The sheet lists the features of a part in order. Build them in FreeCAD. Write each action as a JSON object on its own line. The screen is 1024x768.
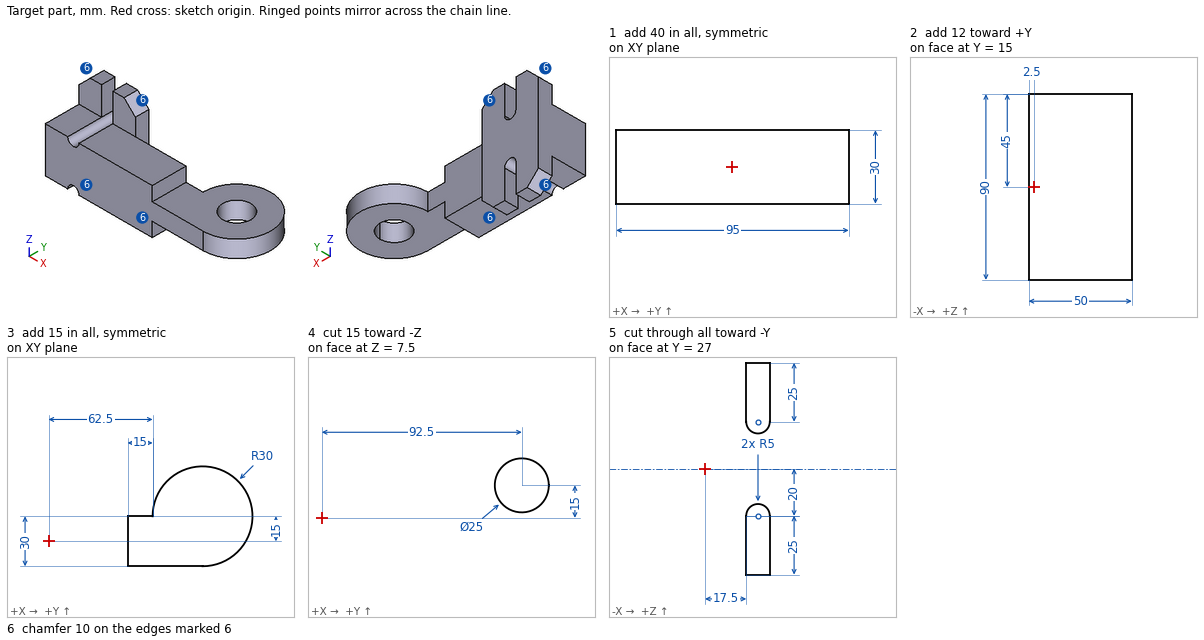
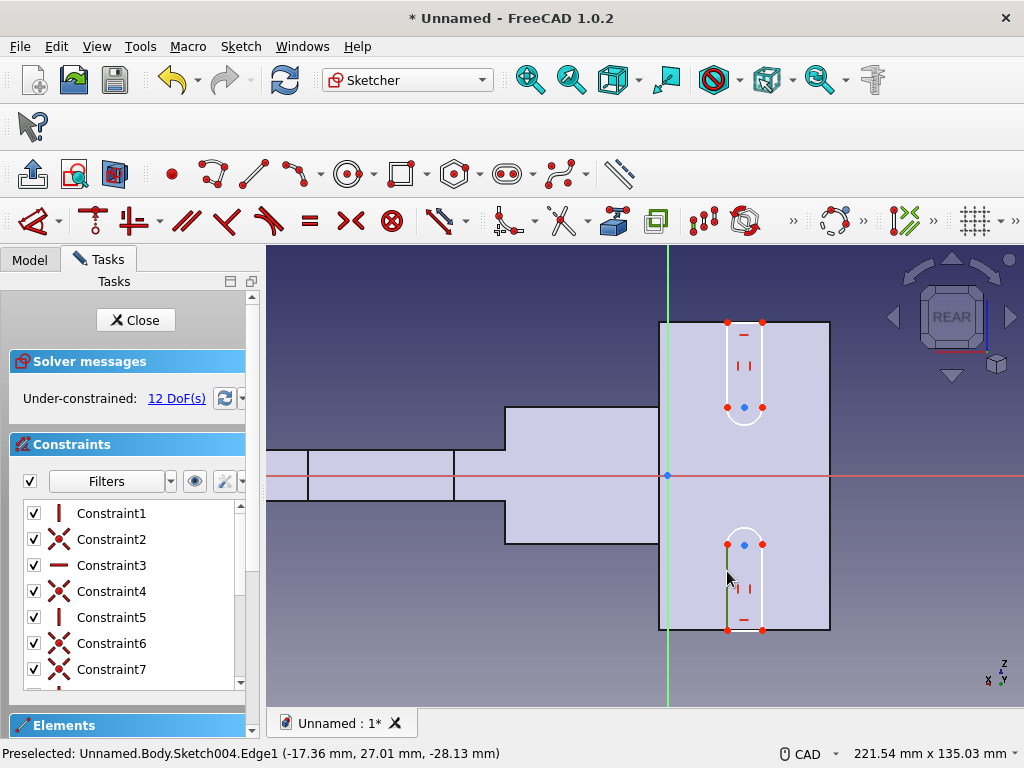
{"action": "left_click", "coordinate": [755, 531]}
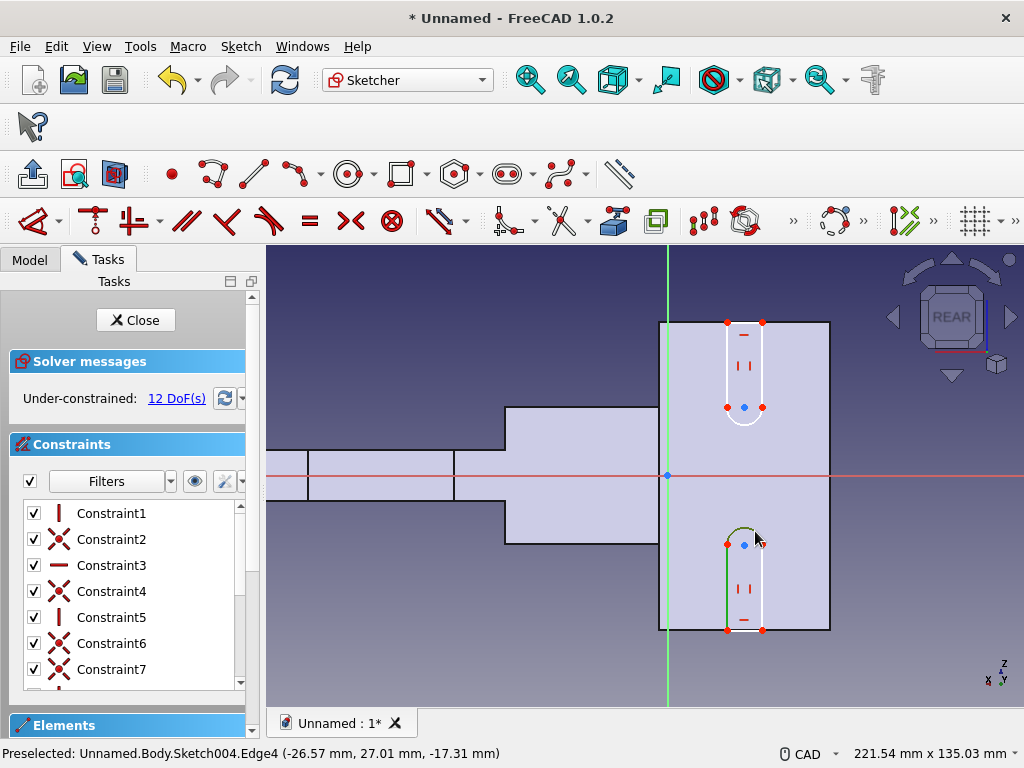
{"action": "left_click", "coordinate": [269, 222]}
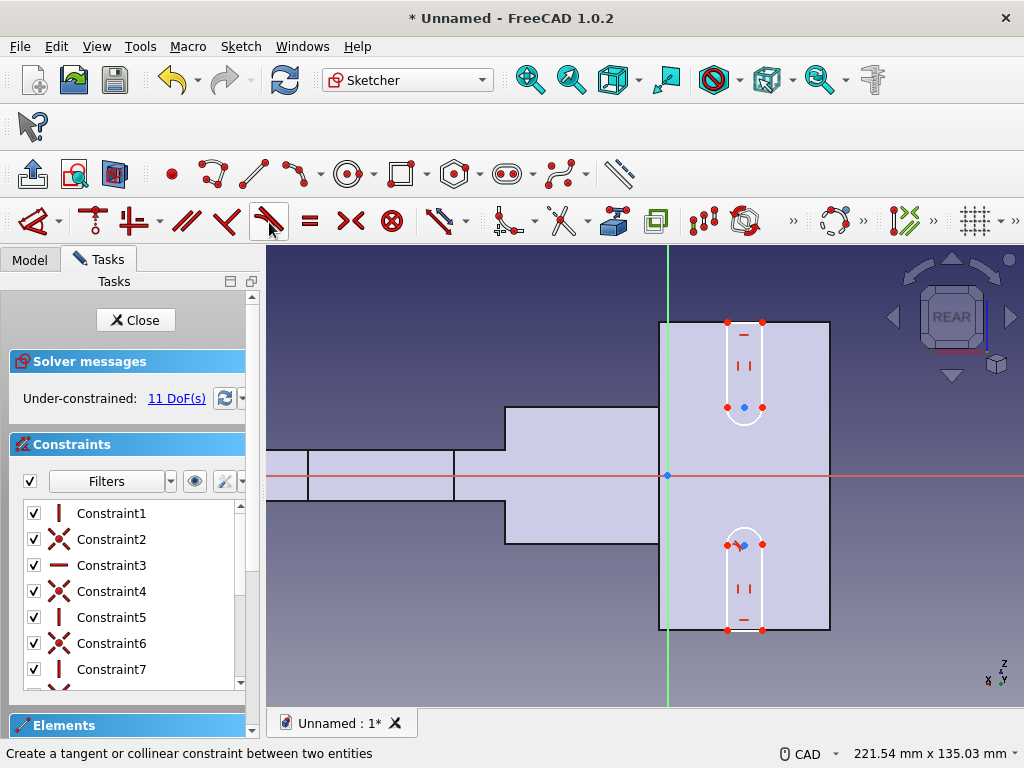
{"action": "left_click", "coordinate": [762, 605]}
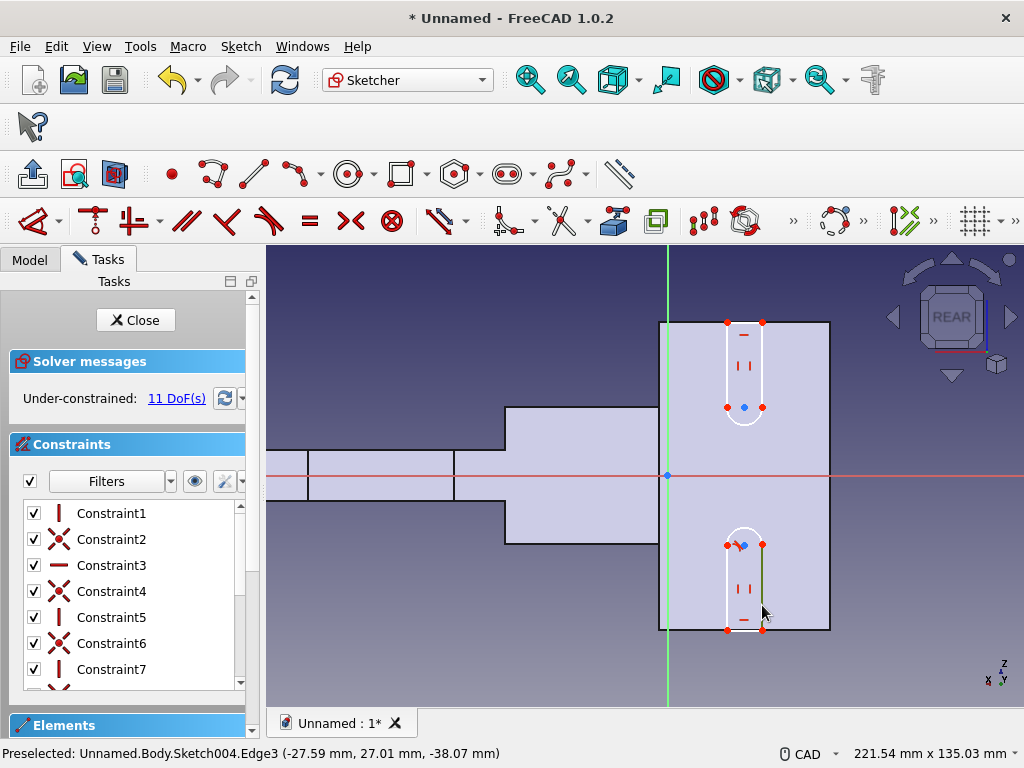
{"action": "left_click", "coordinate": [755, 531]}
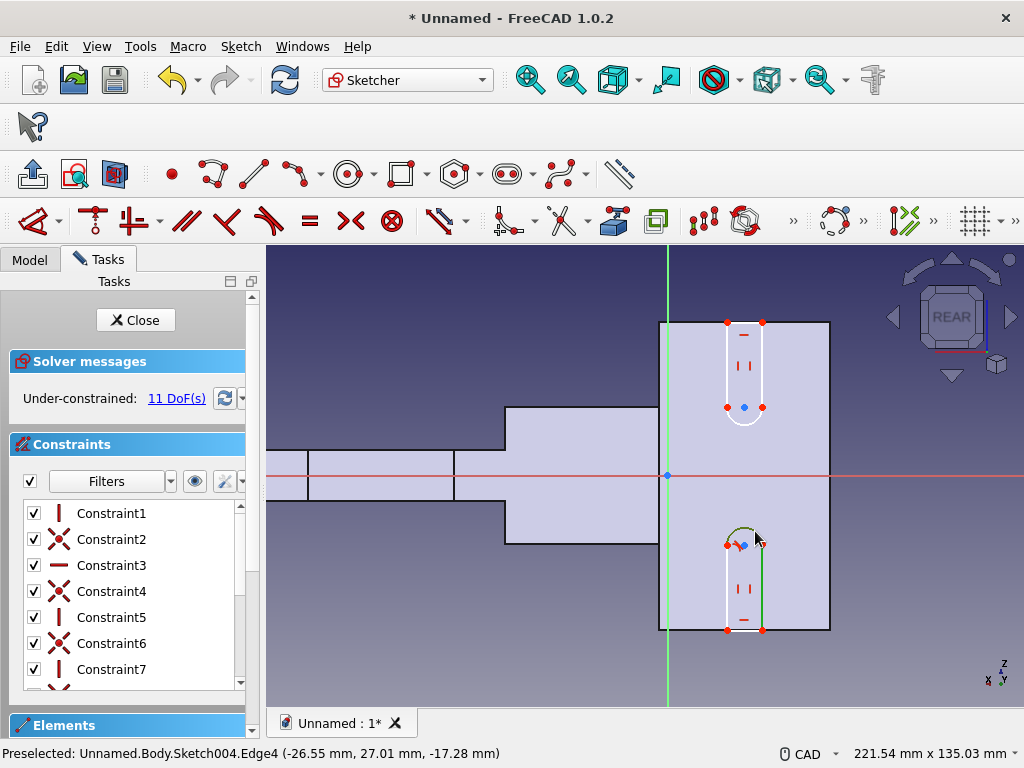
{"action": "left_click", "coordinate": [269, 222]}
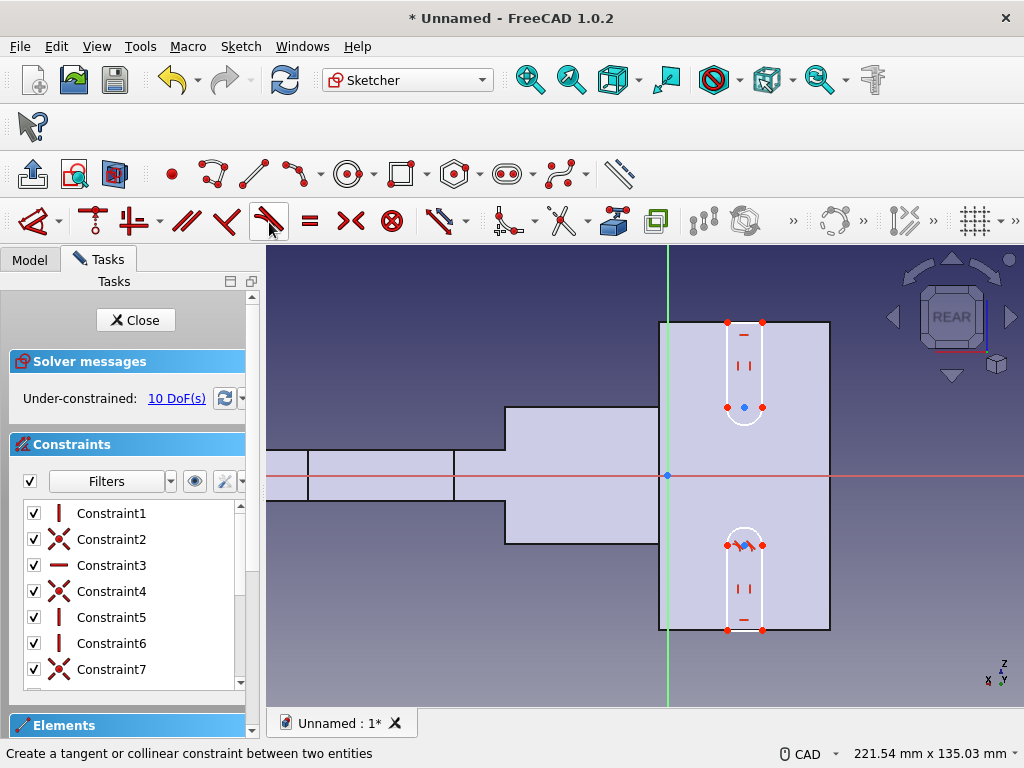
{"action": "left_click", "coordinate": [762, 382]}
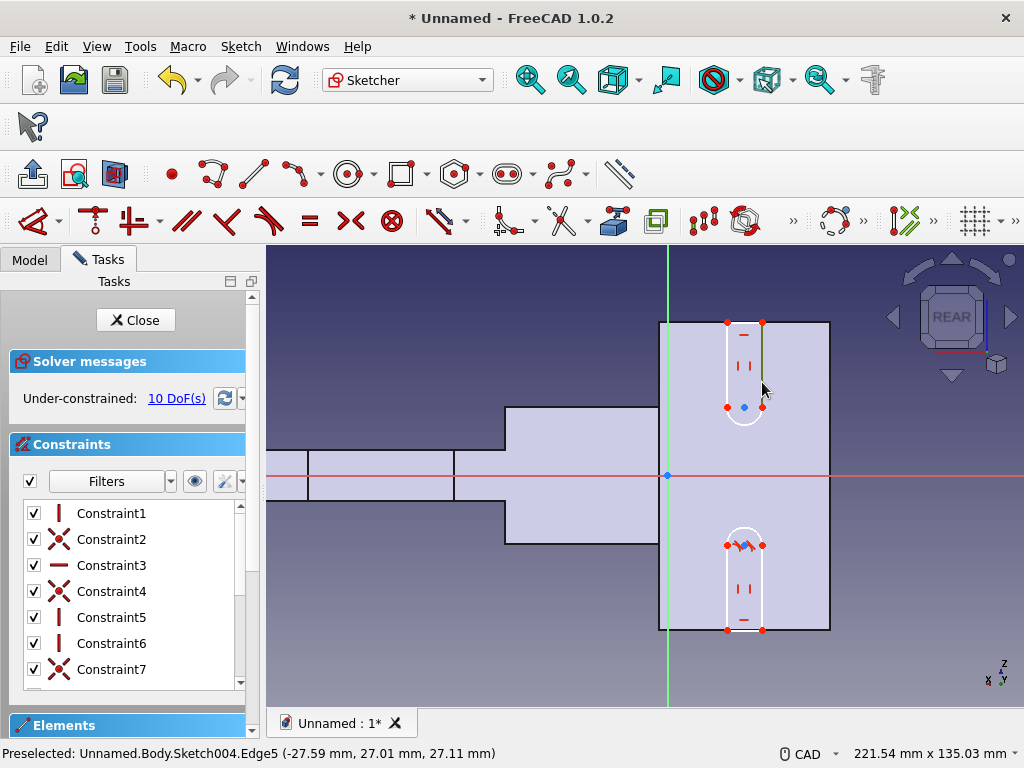
{"action": "left_click", "coordinate": [734, 422]}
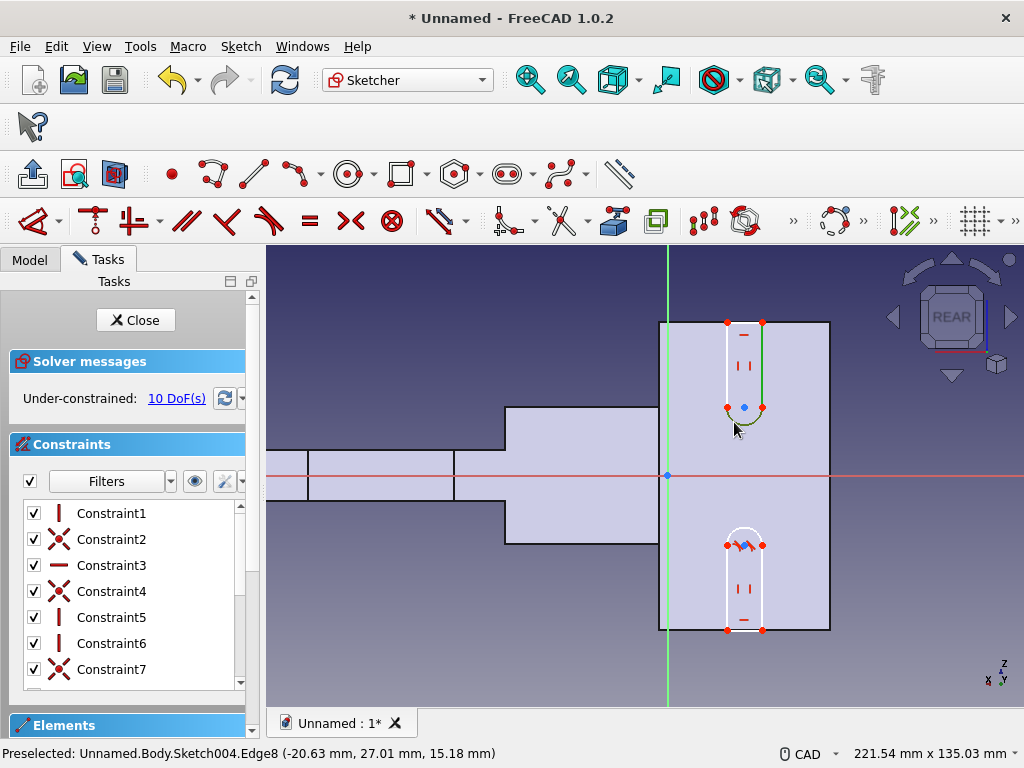
{"action": "left_click", "coordinate": [269, 222]}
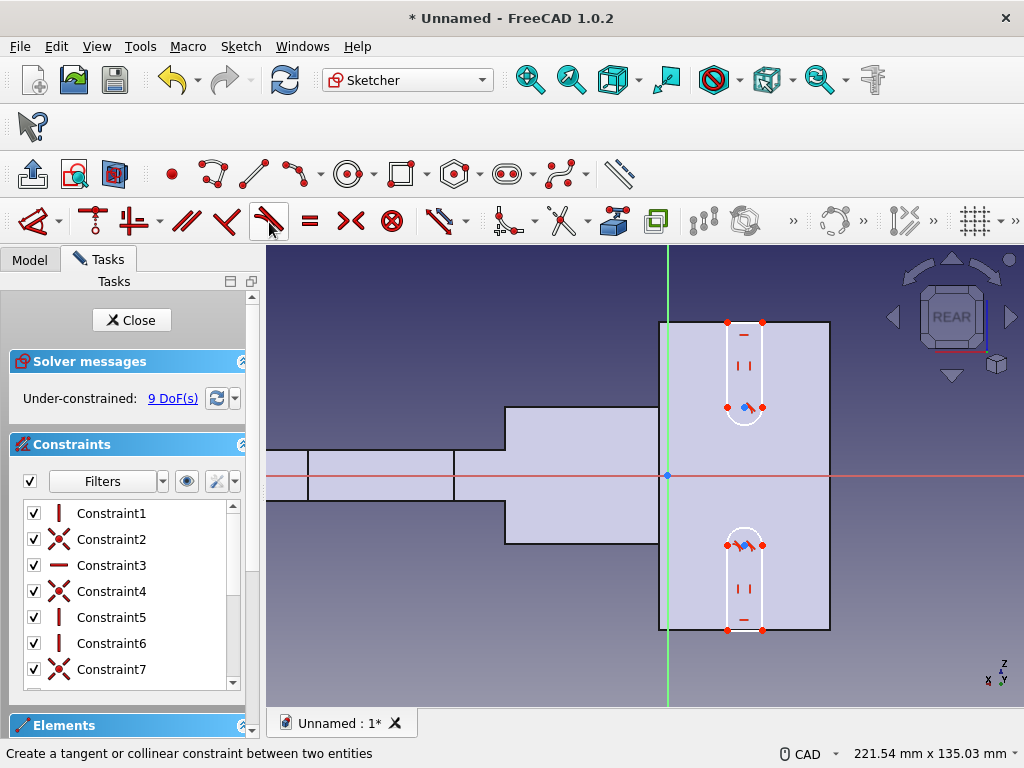
{"action": "left_click", "coordinate": [727, 348]}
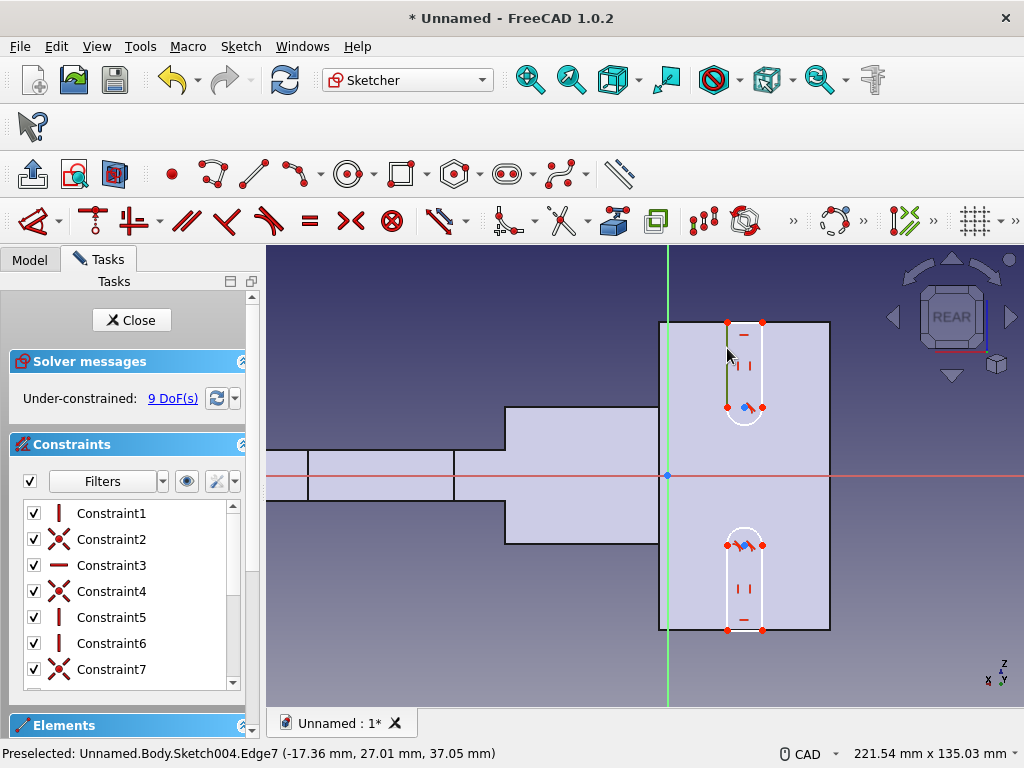
{"action": "left_click", "coordinate": [734, 422]}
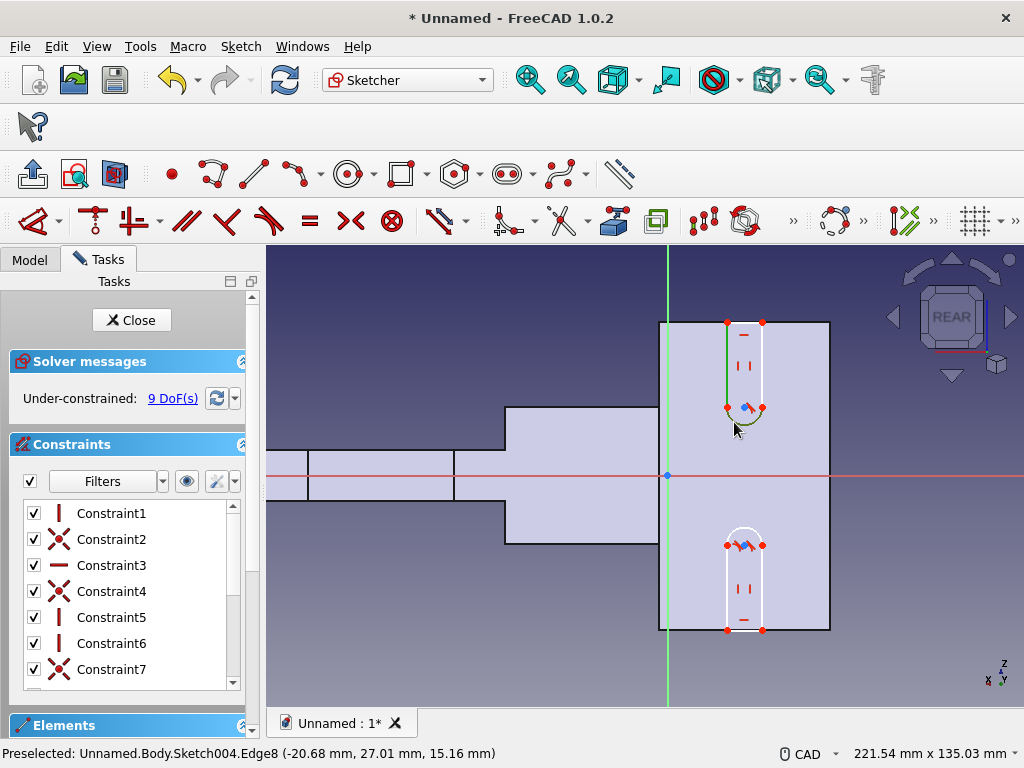
{"action": "left_click", "coordinate": [269, 222]}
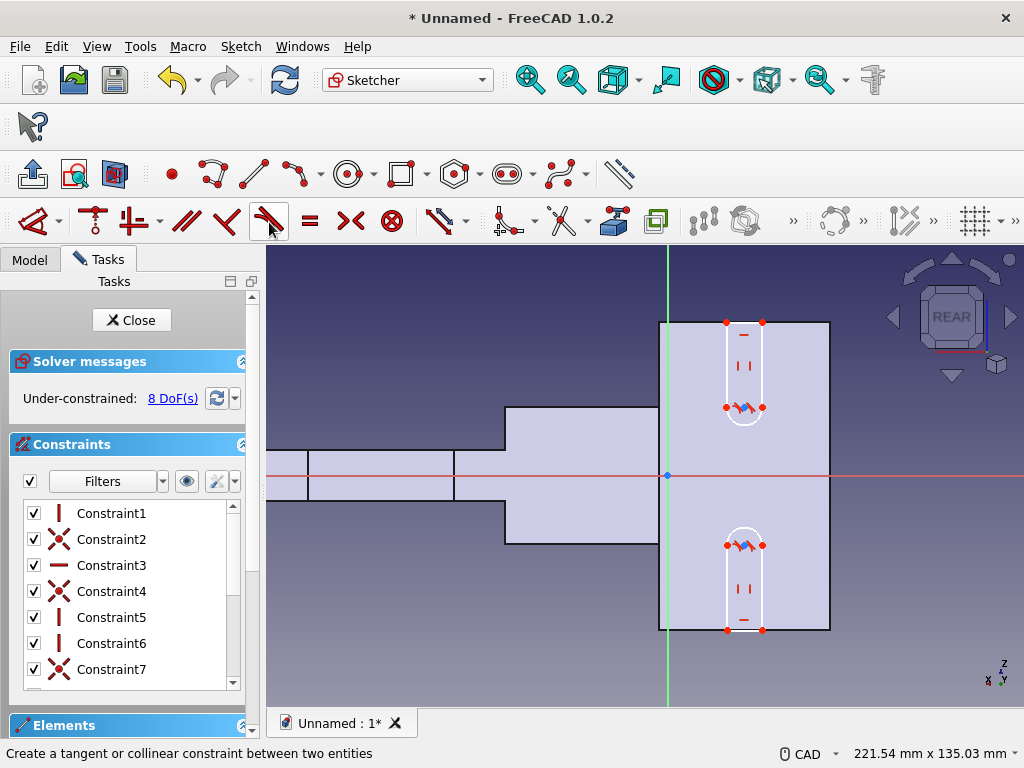
{"action": "left_click", "coordinate": [755, 531]}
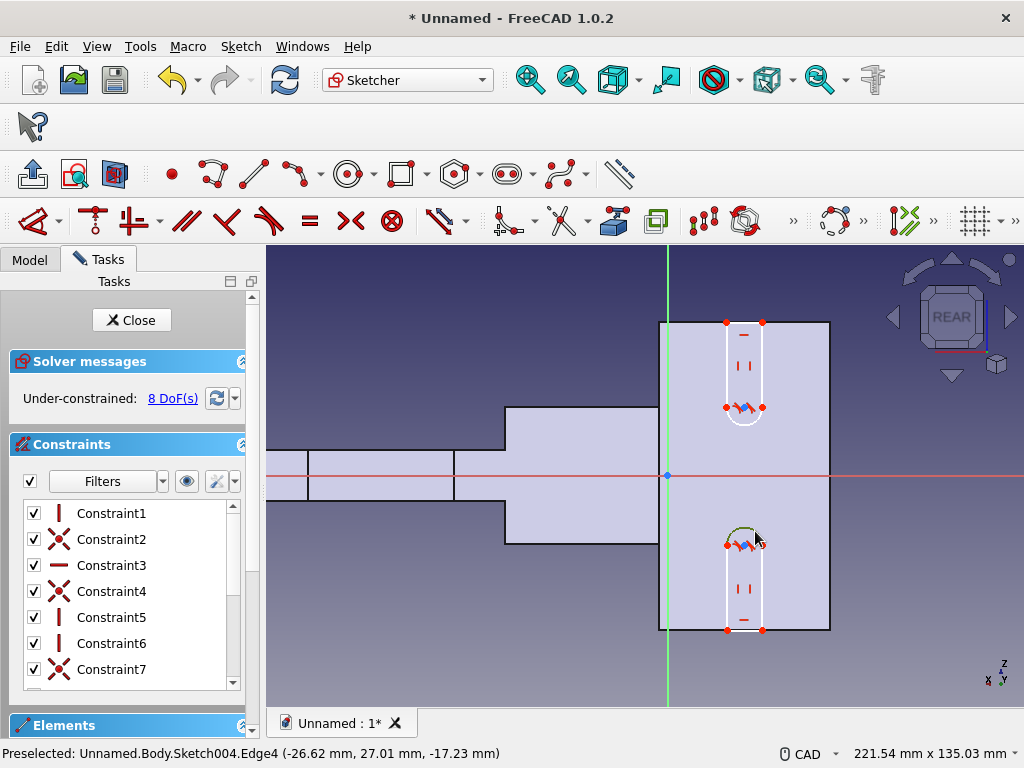
{"action": "left_click", "coordinate": [734, 422]}